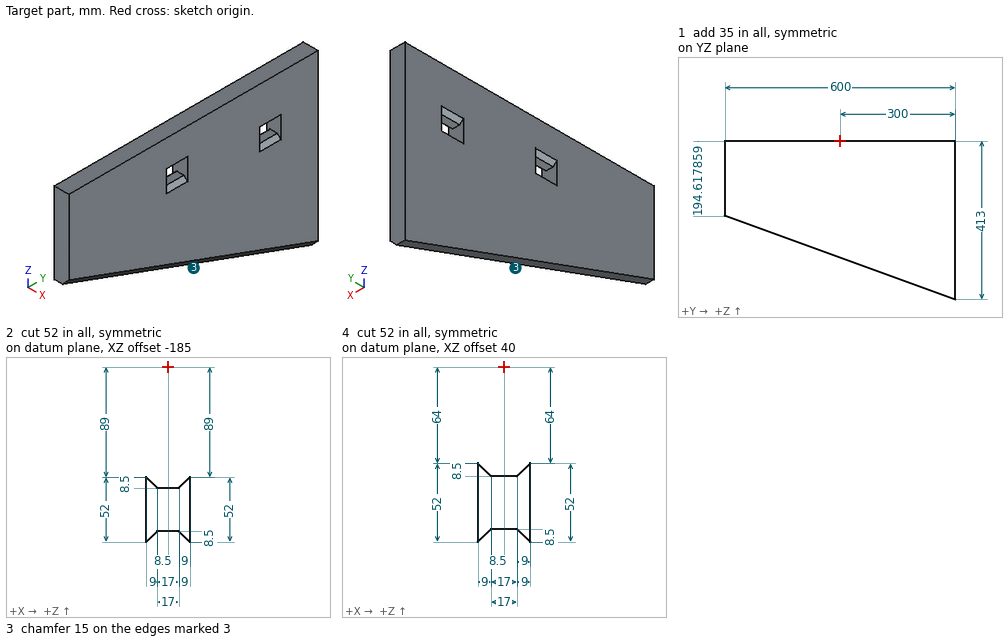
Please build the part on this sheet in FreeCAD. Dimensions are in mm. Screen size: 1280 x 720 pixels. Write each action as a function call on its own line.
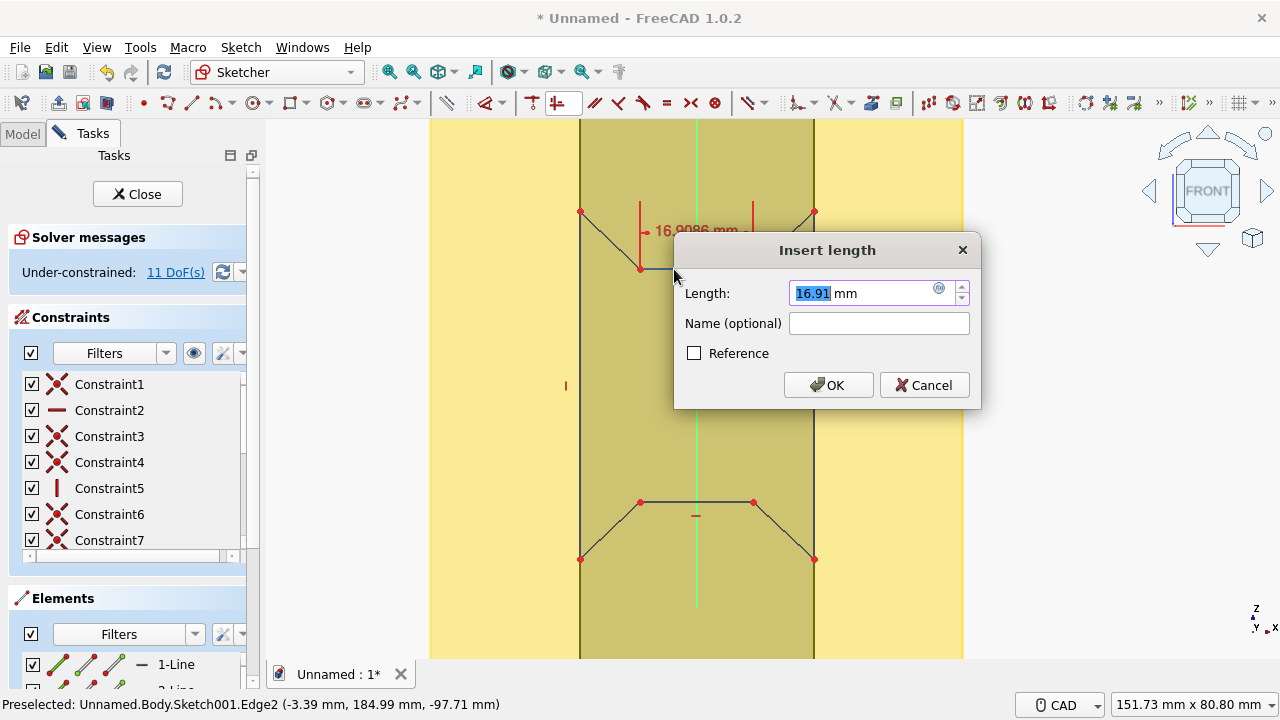
text(17)
key(Return)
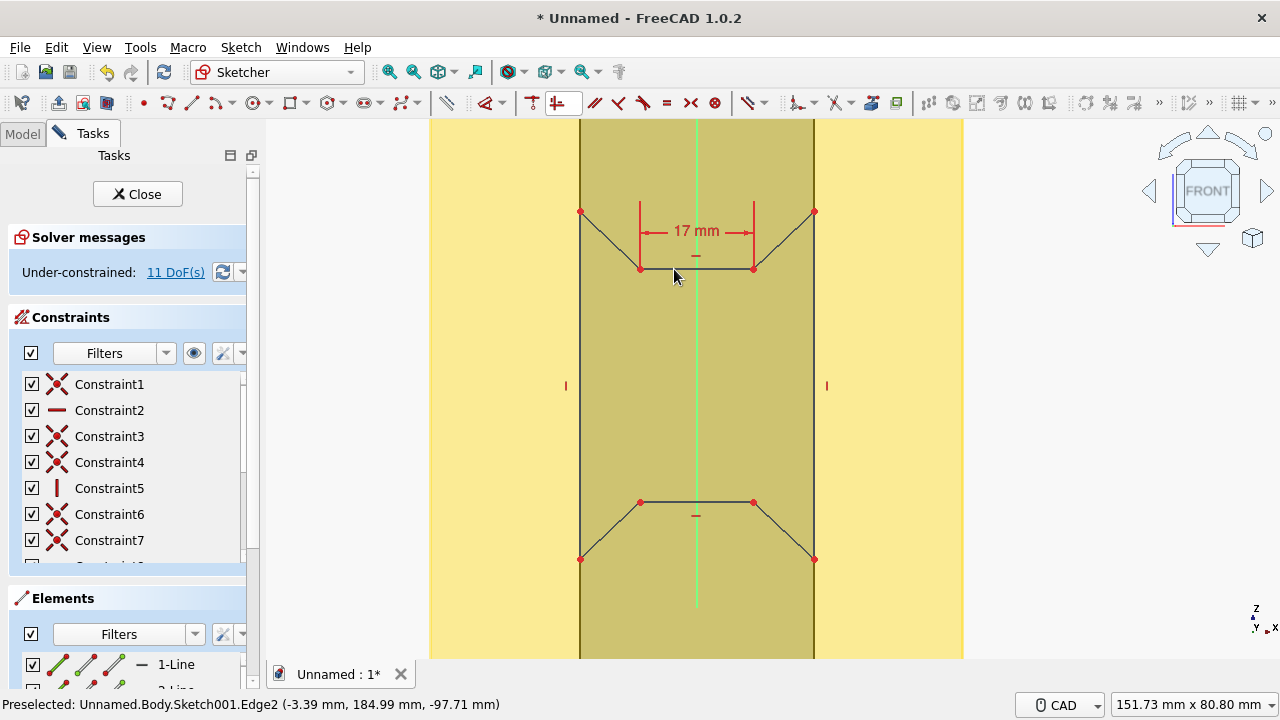
click(814, 316)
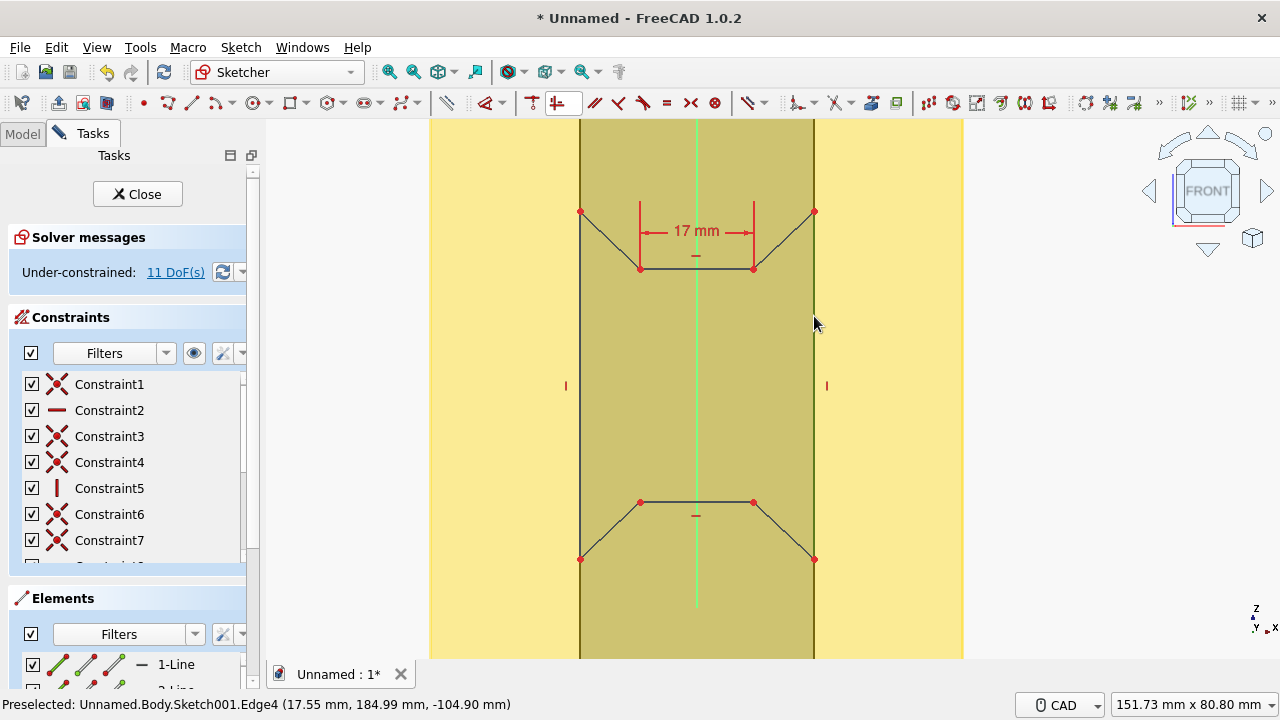
click(504, 104)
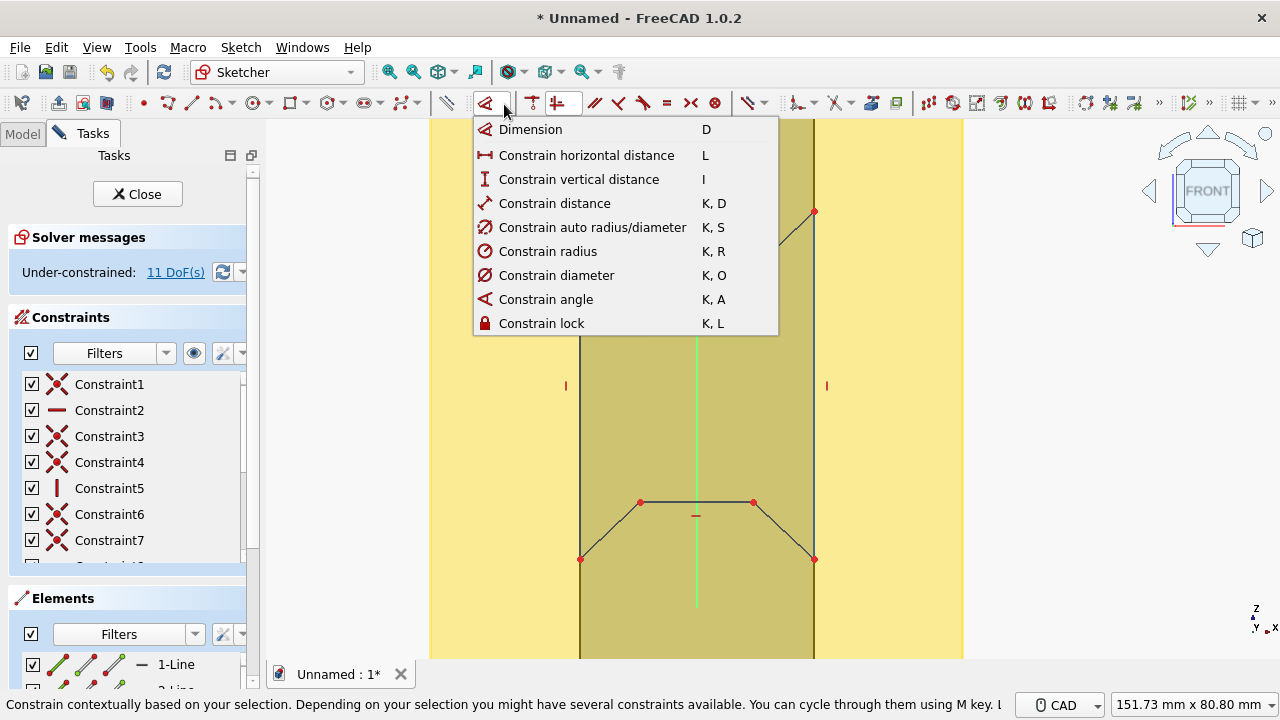
click(626, 179)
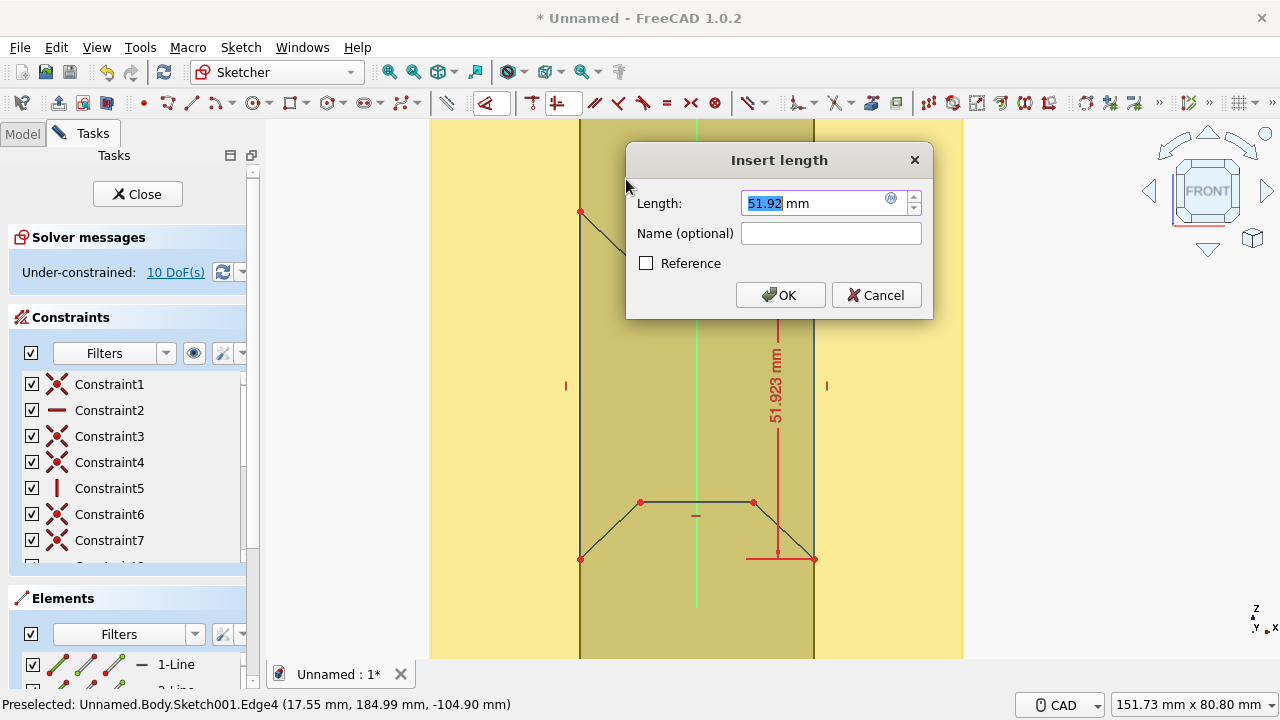
text(52)
key(Return)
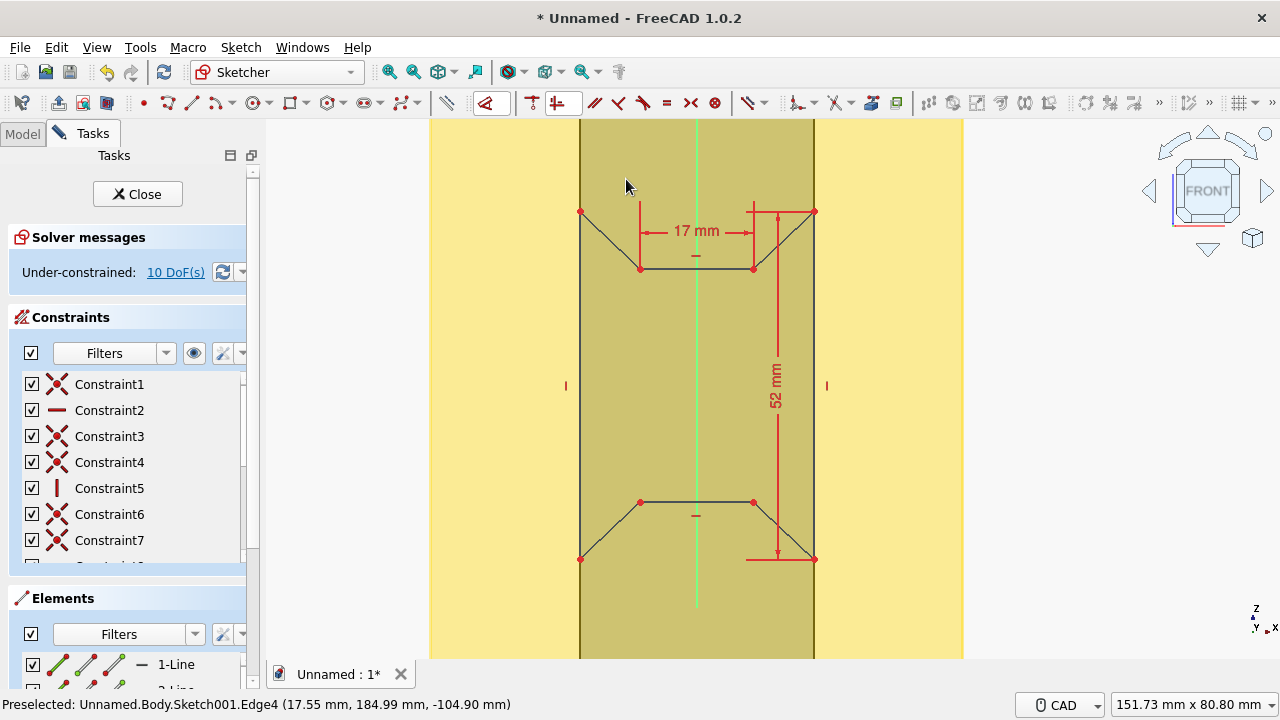
click(719, 502)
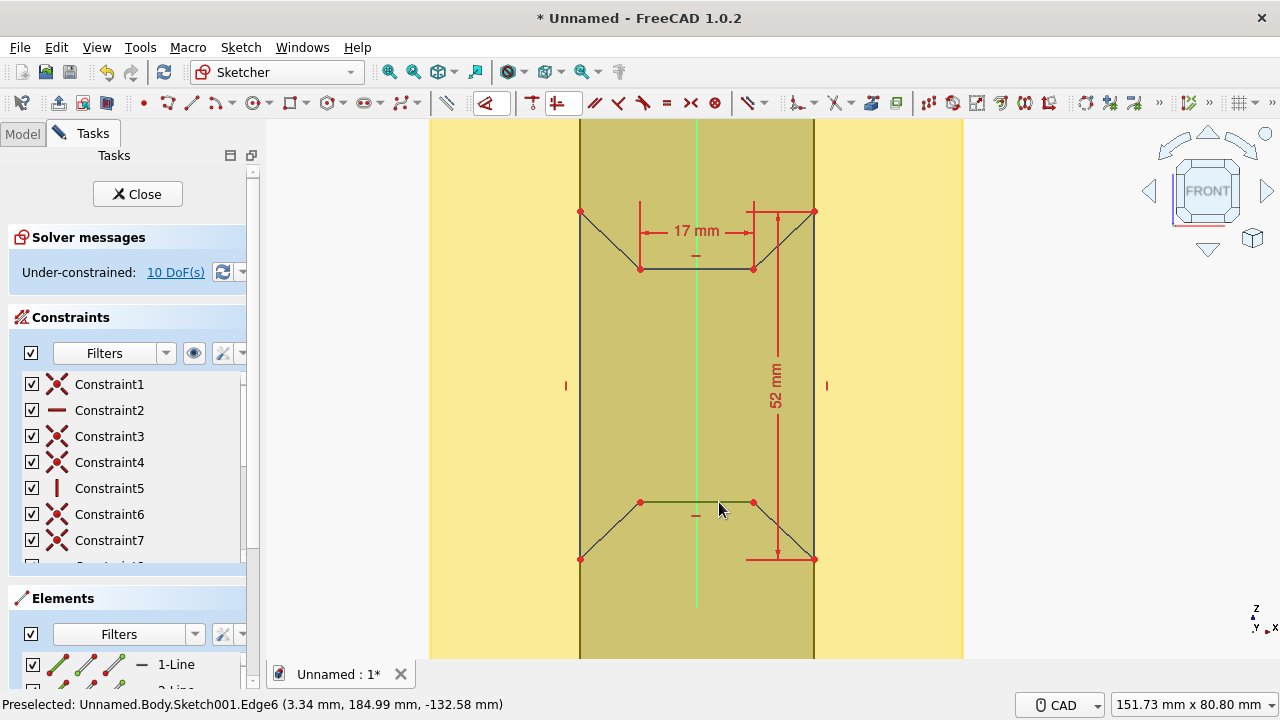
click(504, 104)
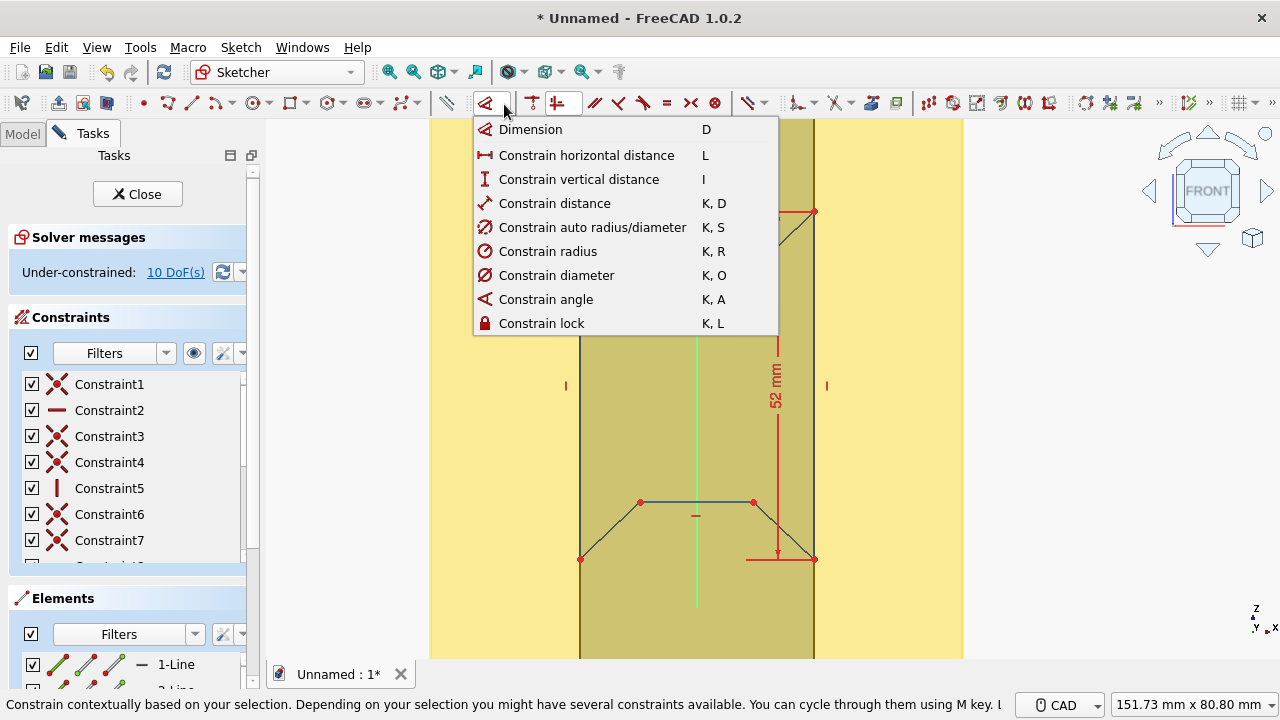
click(626, 155)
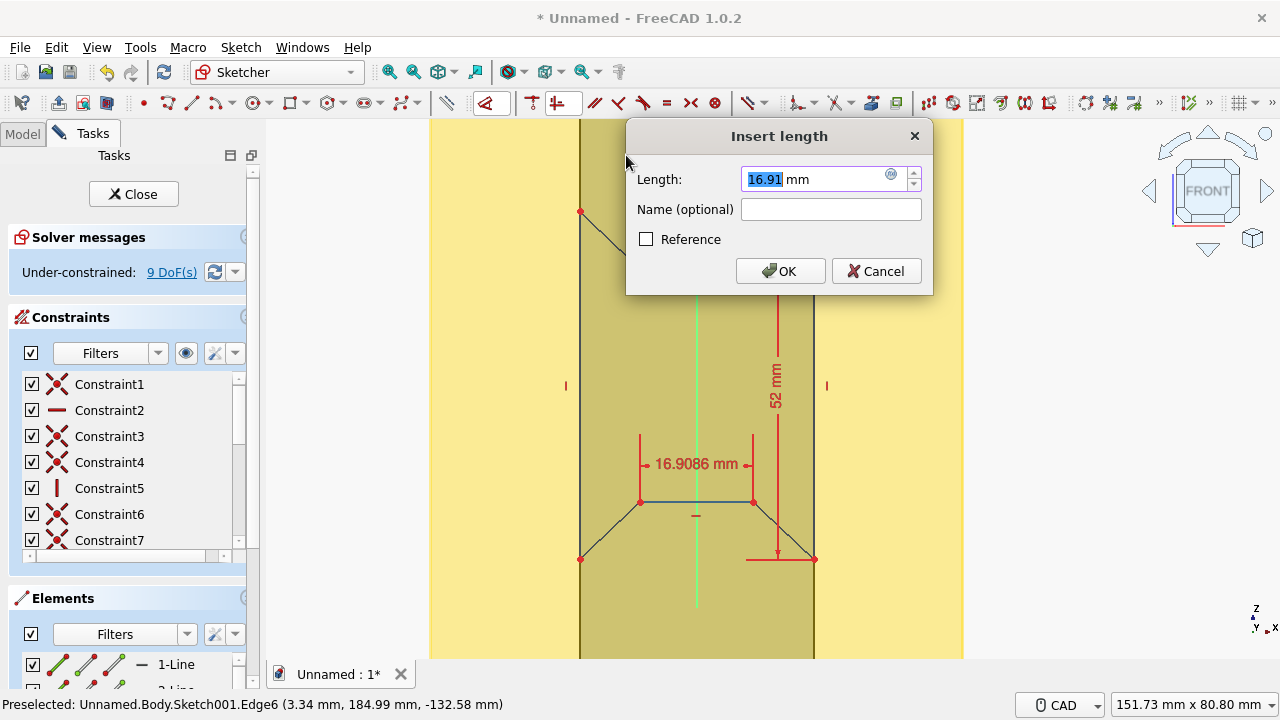
text(17)
key(Return)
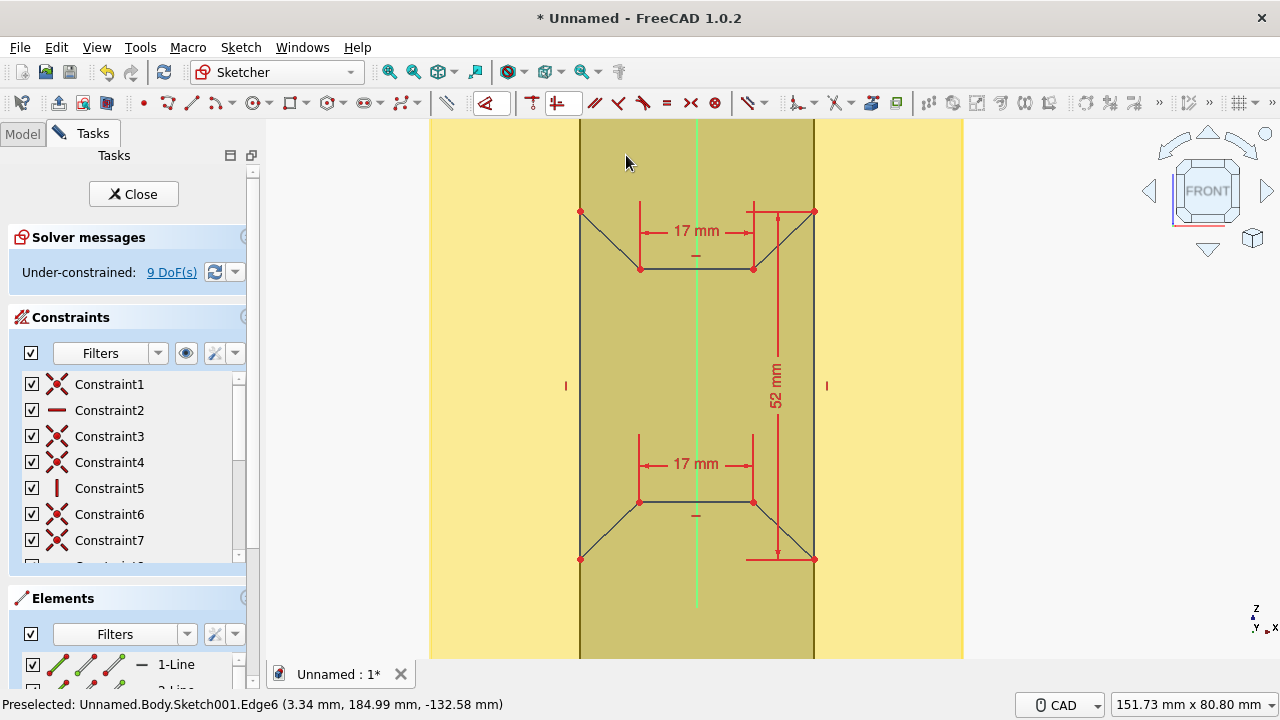
click(580, 455)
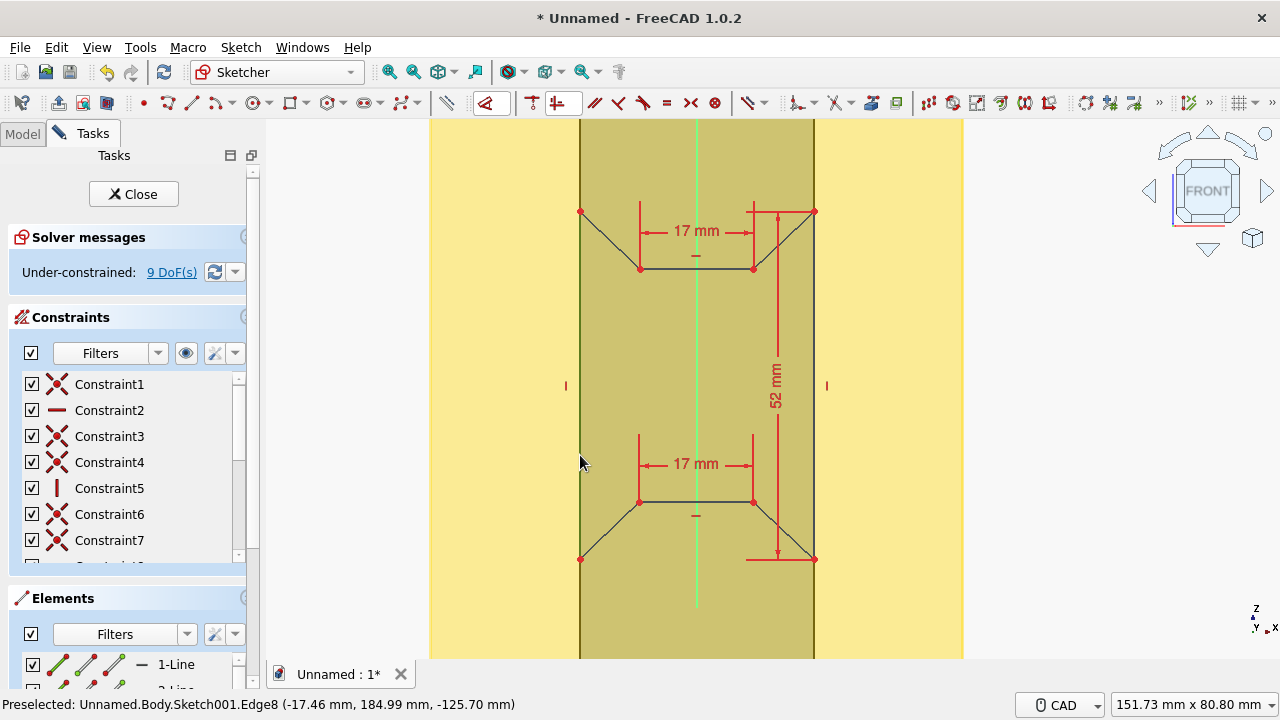
key(i)